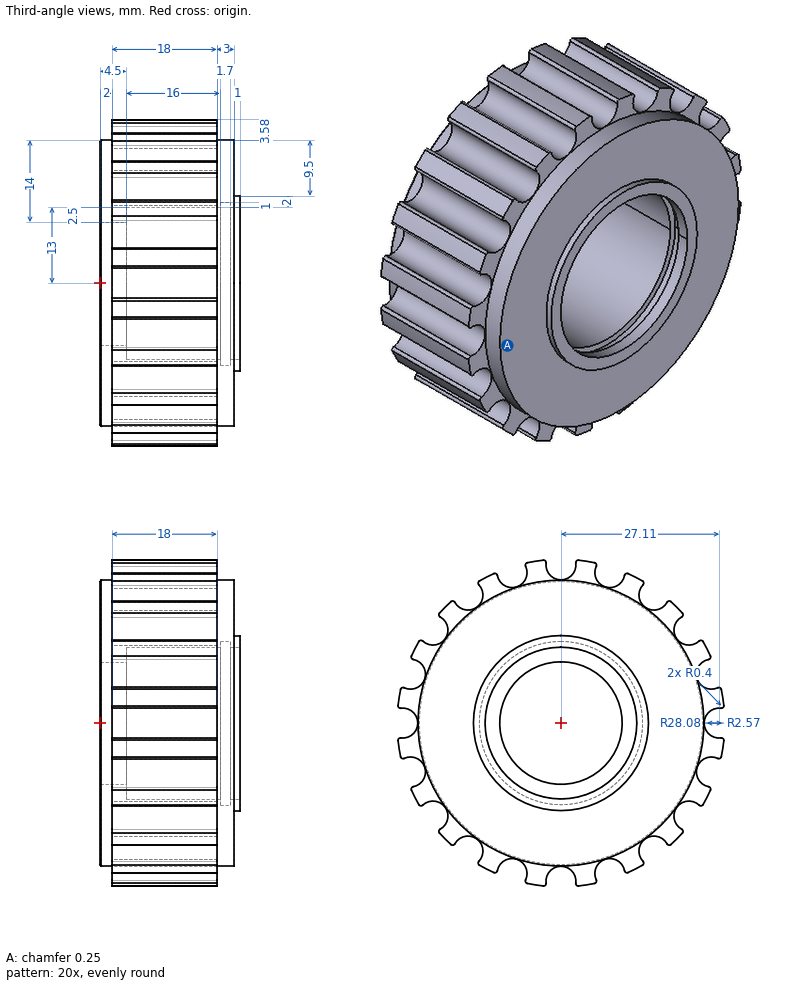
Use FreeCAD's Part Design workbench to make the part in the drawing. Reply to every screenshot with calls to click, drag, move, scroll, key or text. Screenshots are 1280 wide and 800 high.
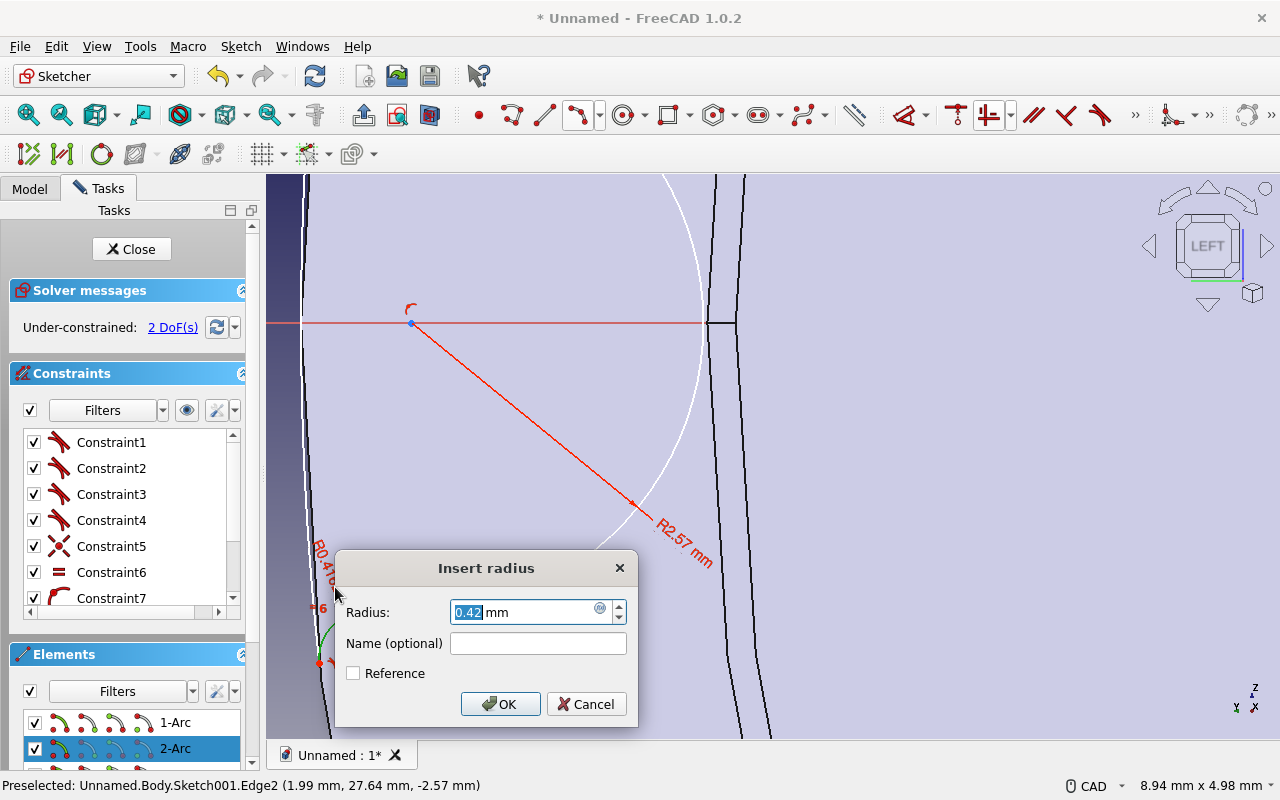
text(0.4)
key(Return)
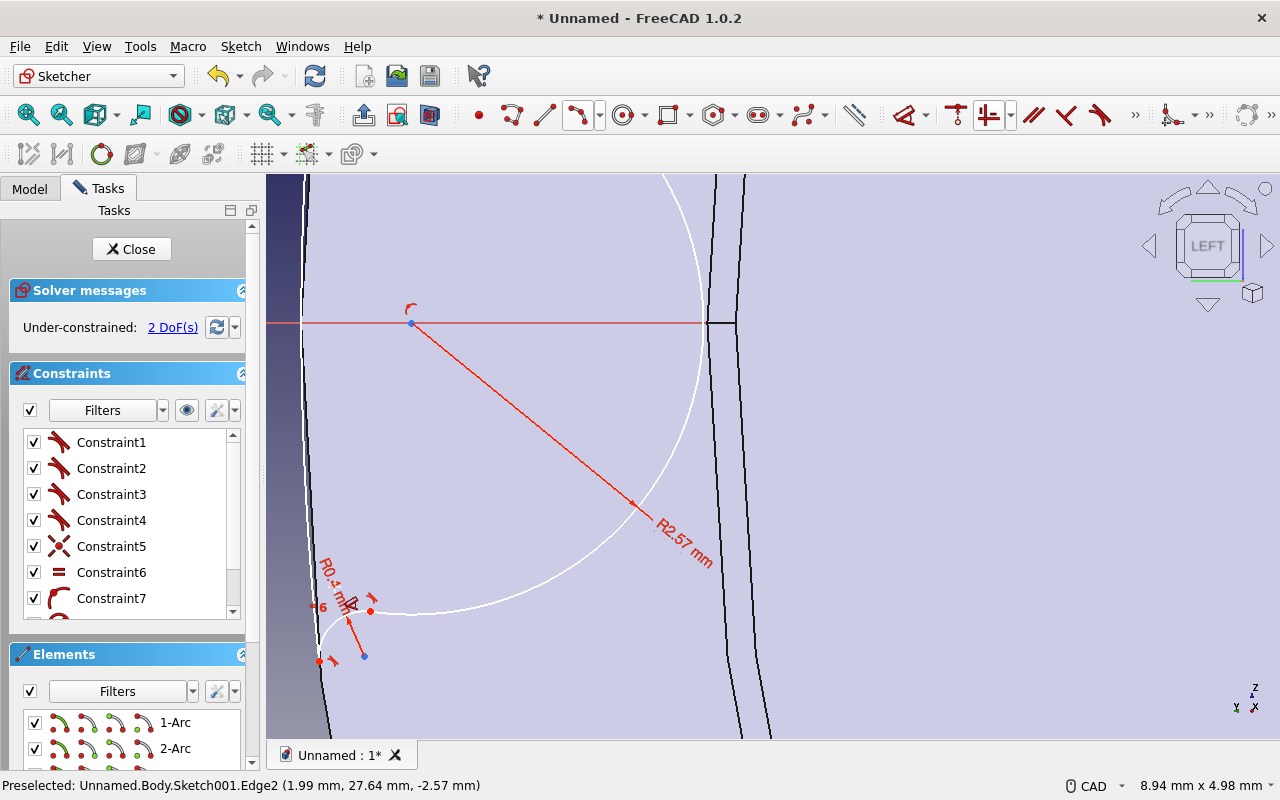
click(304, 459)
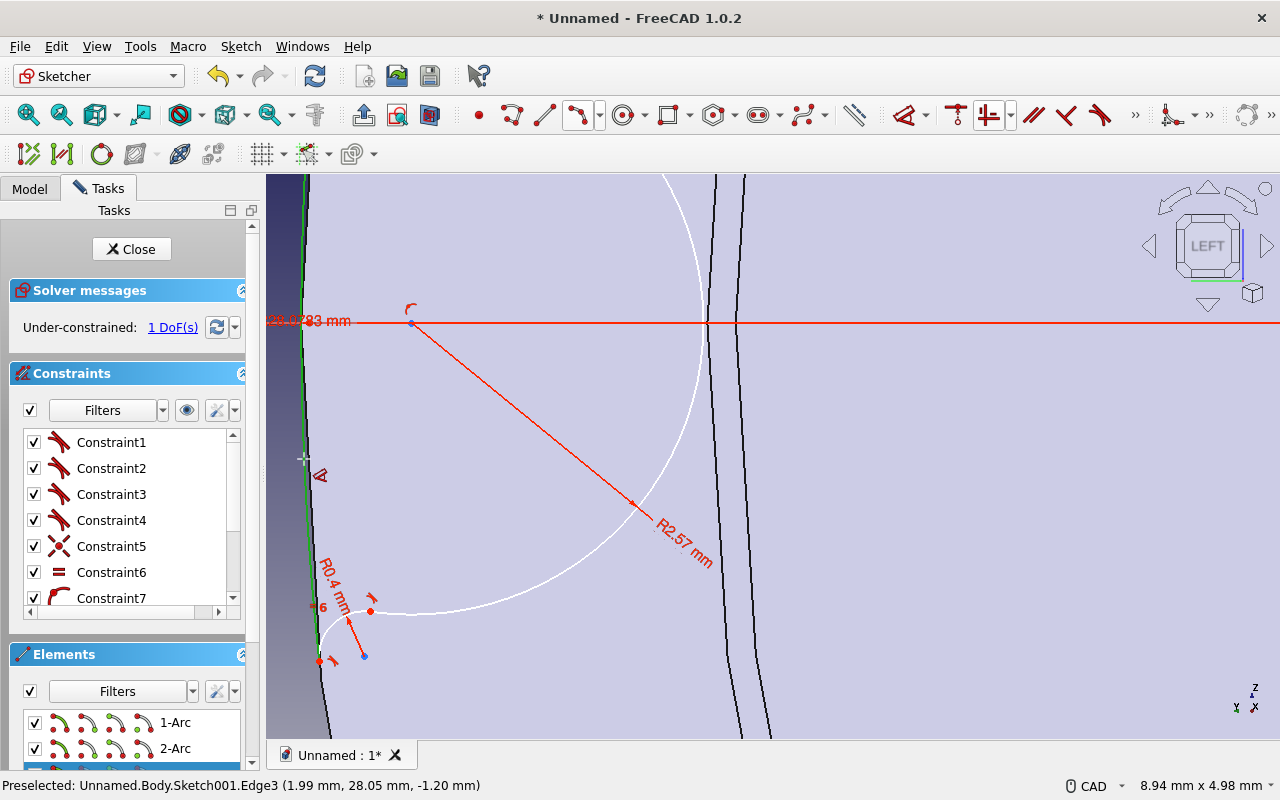
key(Escape)
key(Escape)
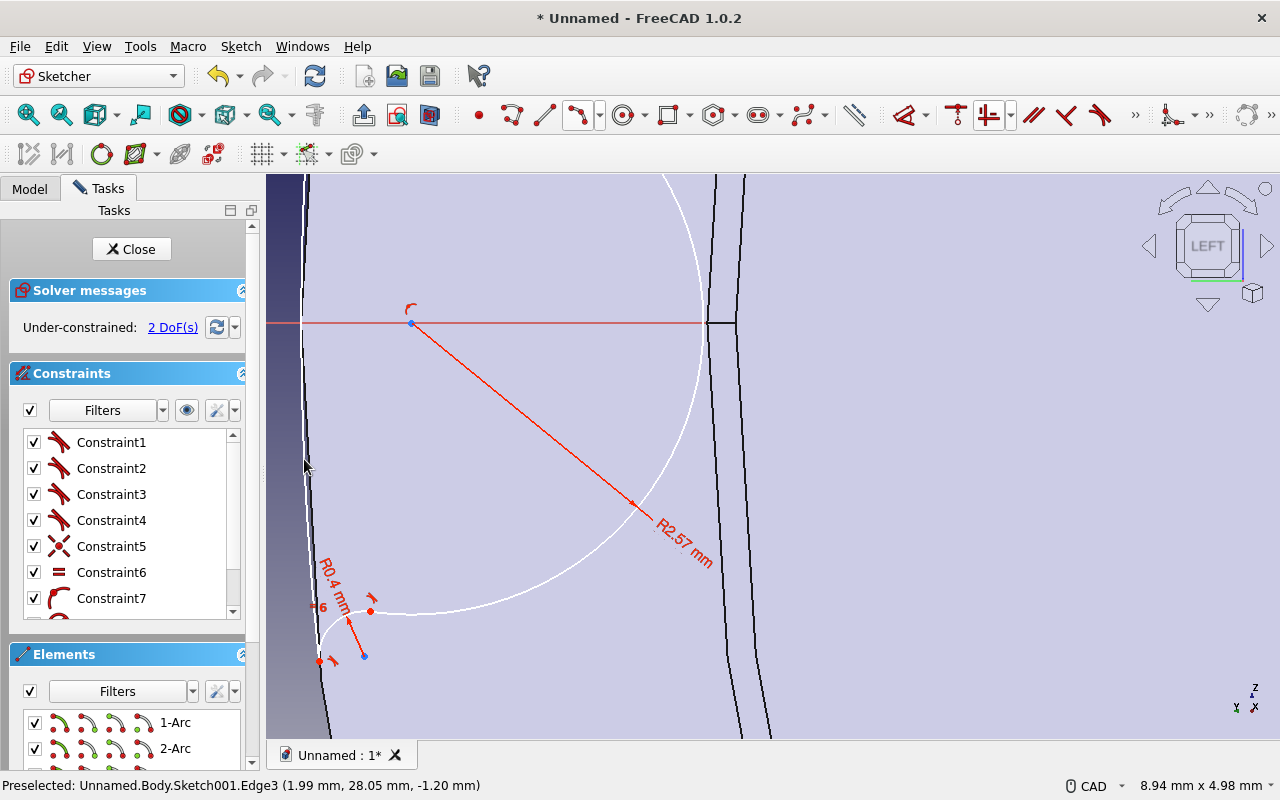
click(304, 459)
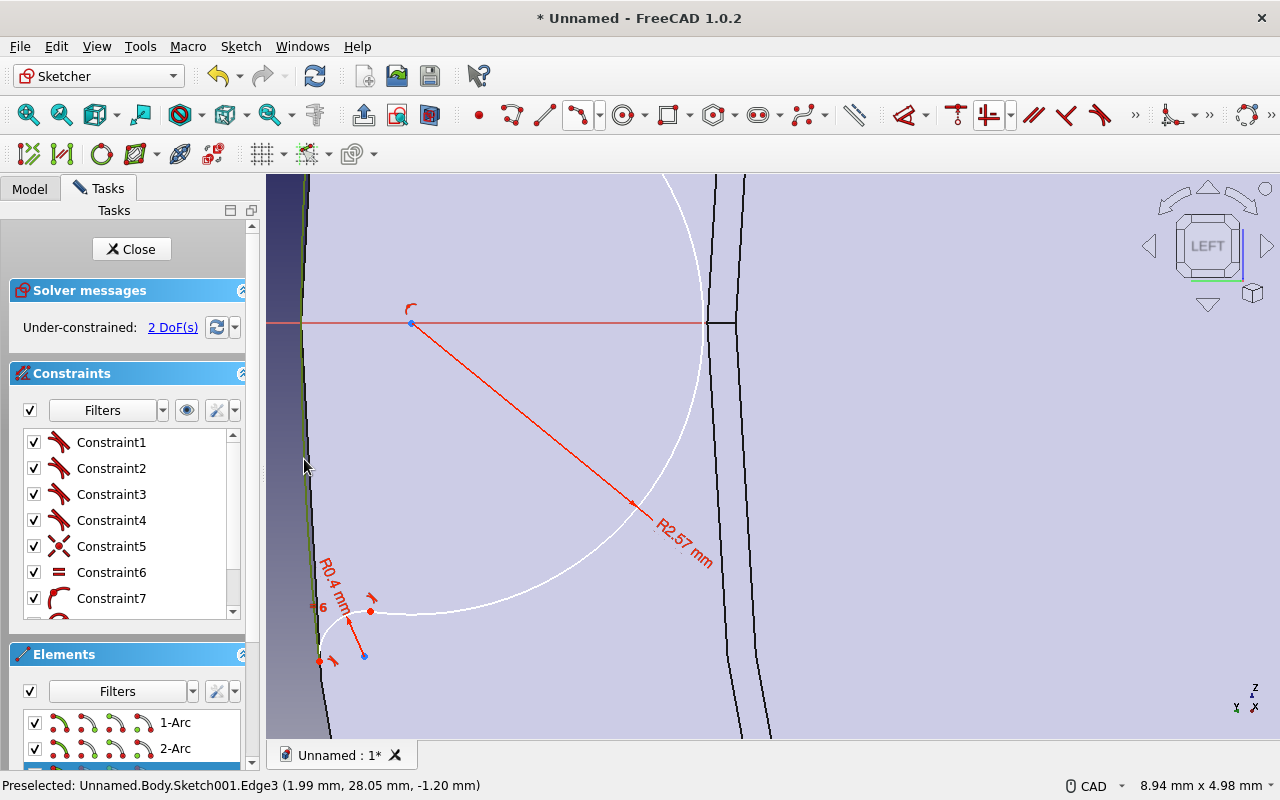
click(926, 116)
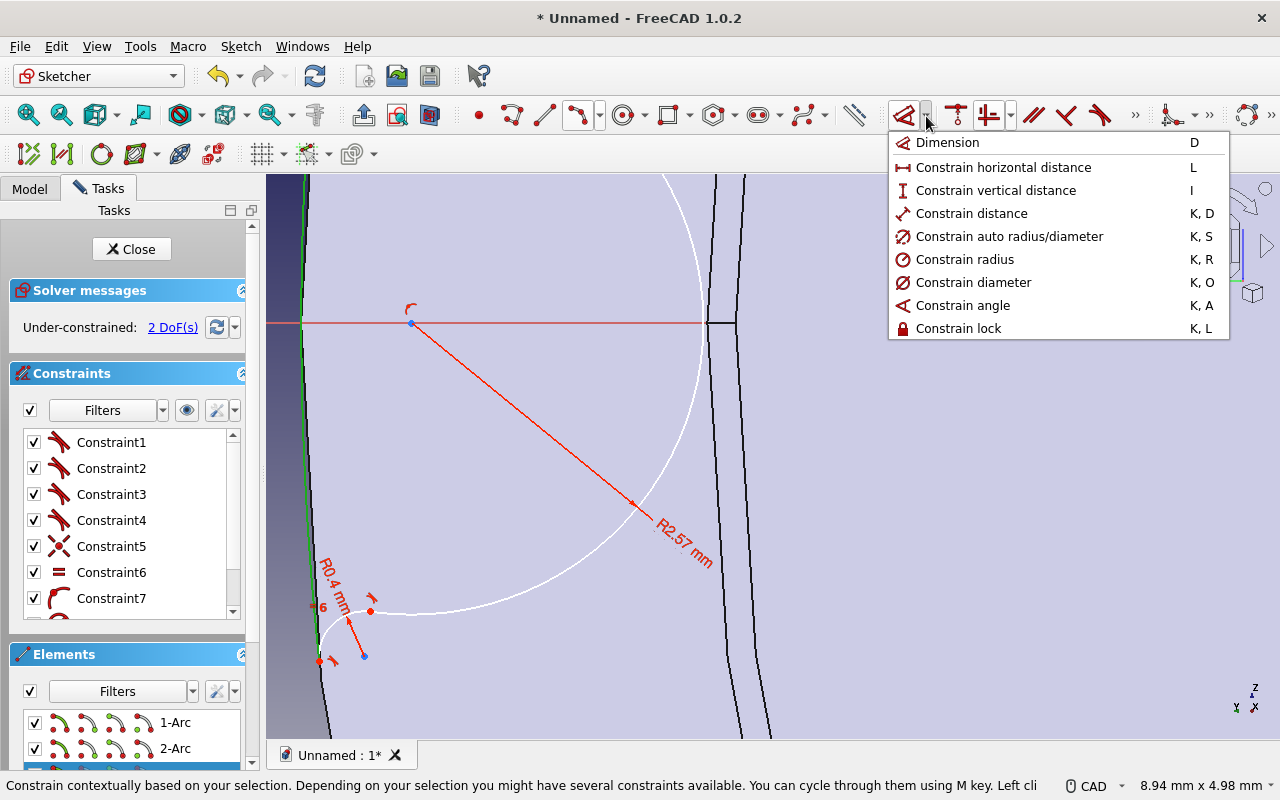
click(1059, 260)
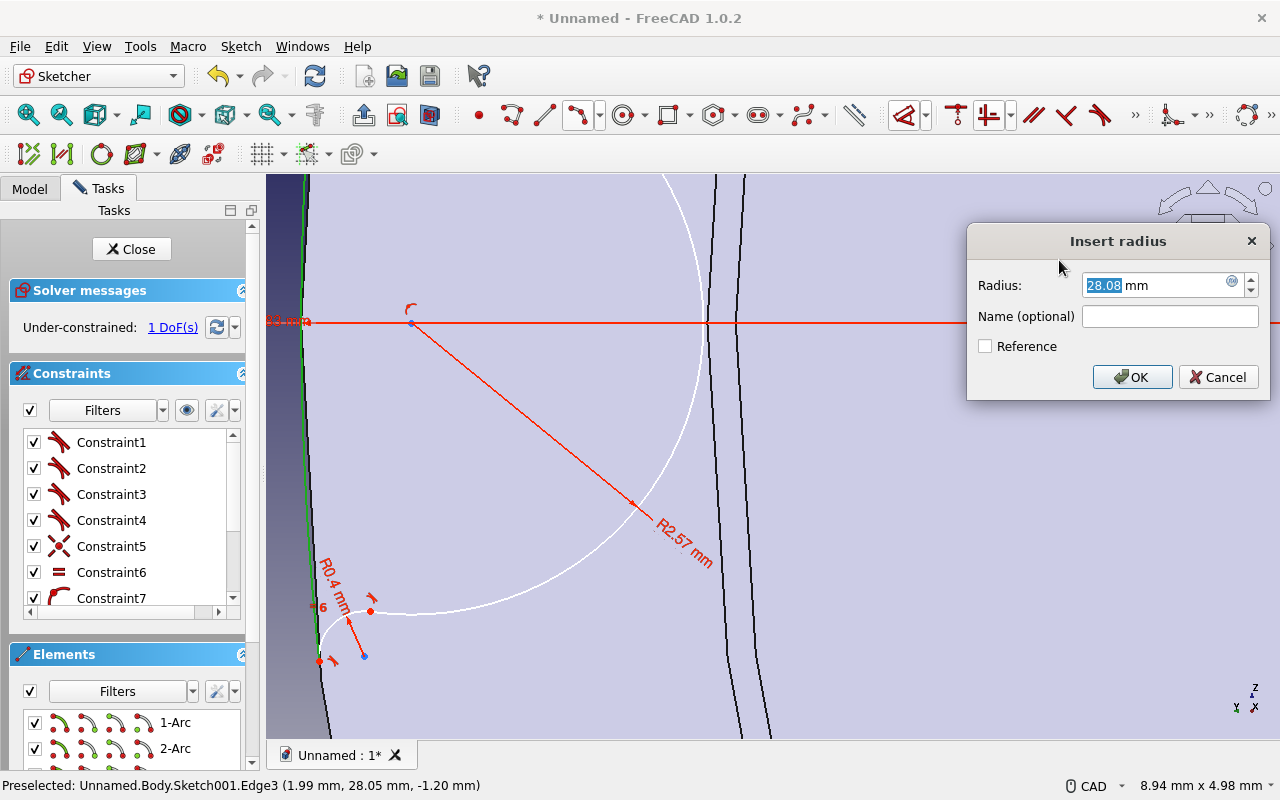
text(28.08)
key(Return)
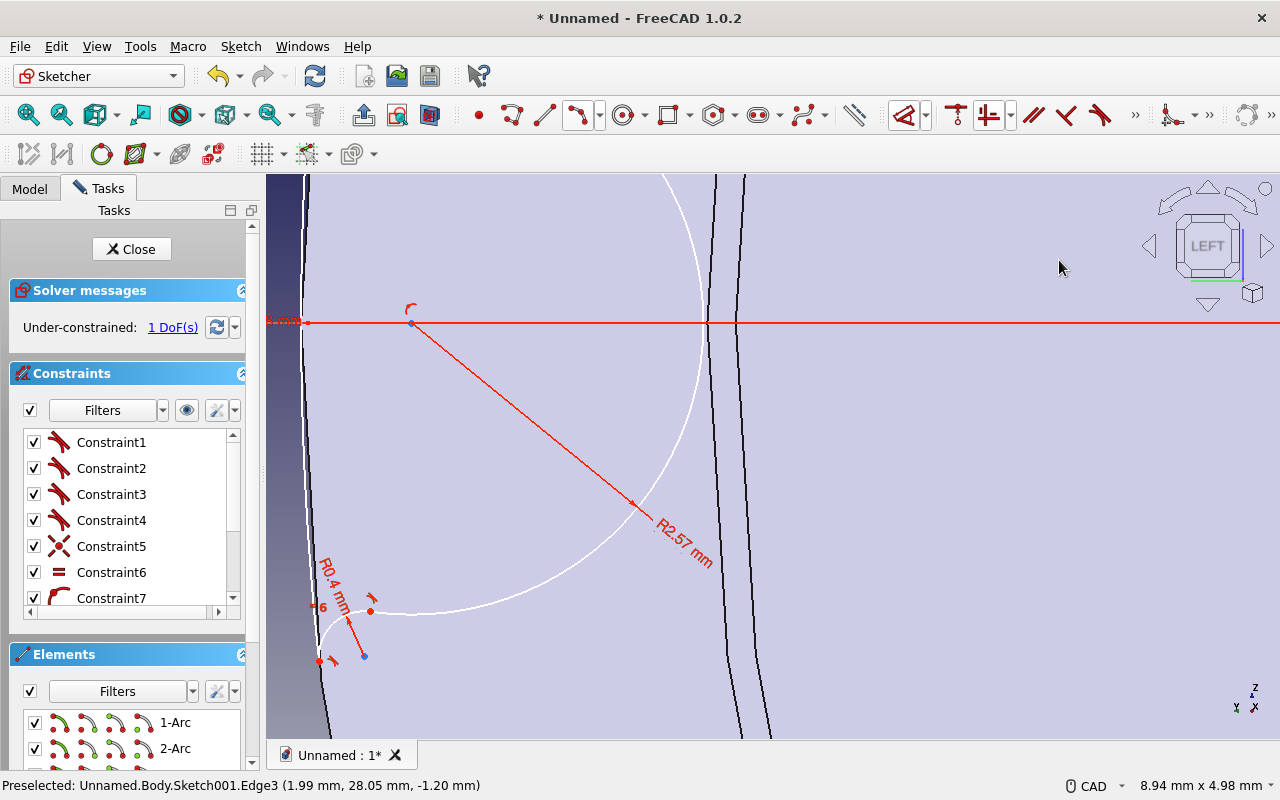
click(412, 323)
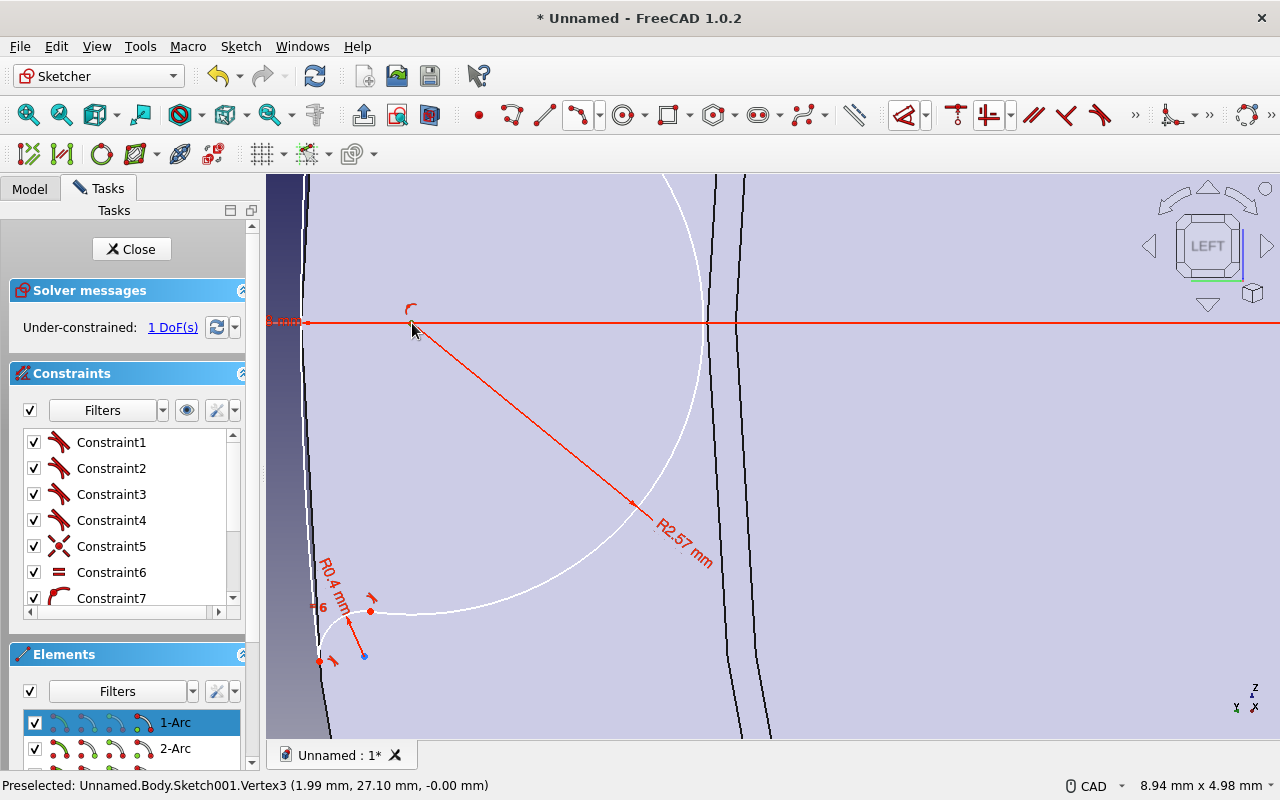
click(926, 116)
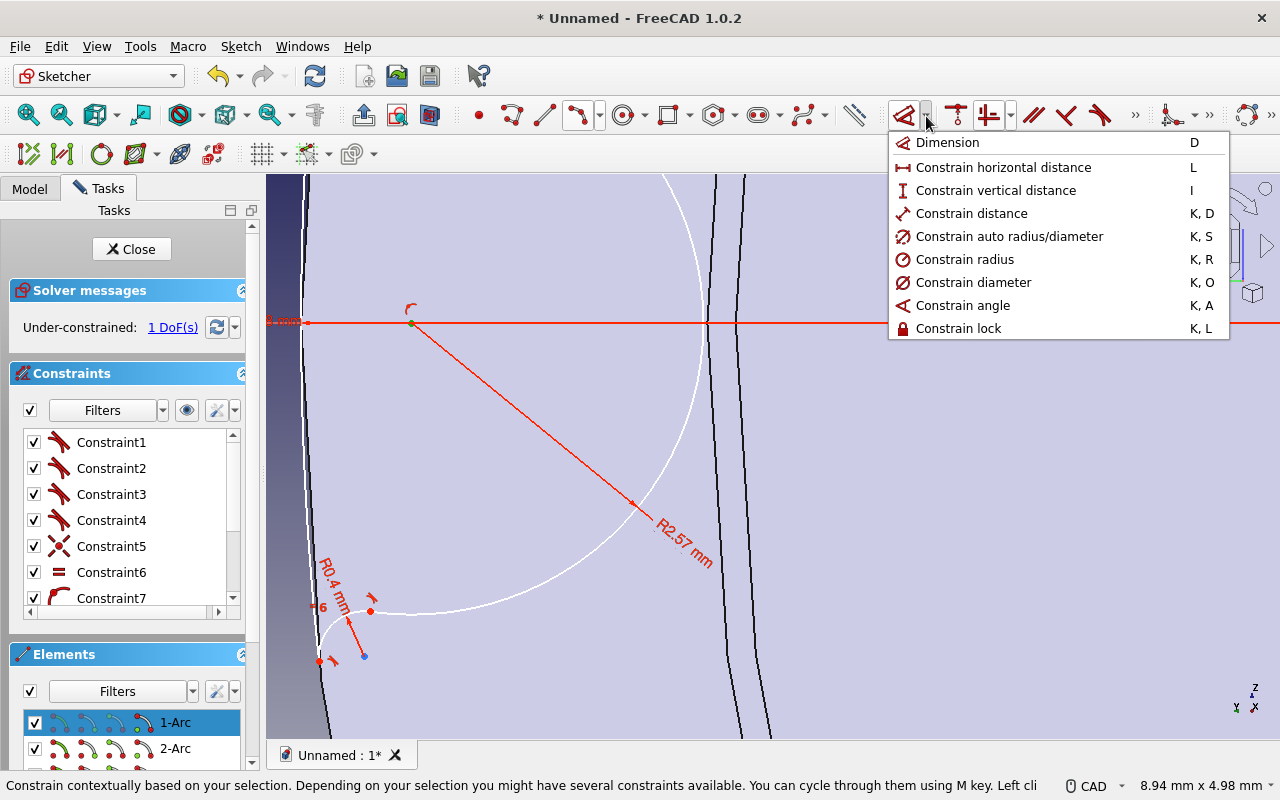
click(1059, 168)